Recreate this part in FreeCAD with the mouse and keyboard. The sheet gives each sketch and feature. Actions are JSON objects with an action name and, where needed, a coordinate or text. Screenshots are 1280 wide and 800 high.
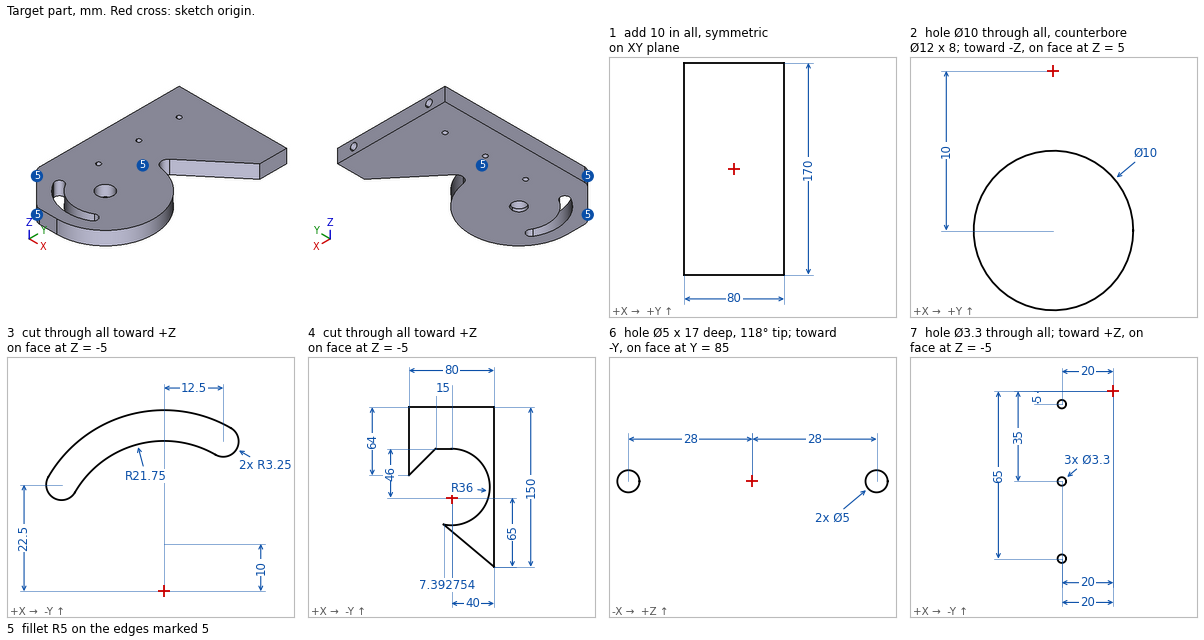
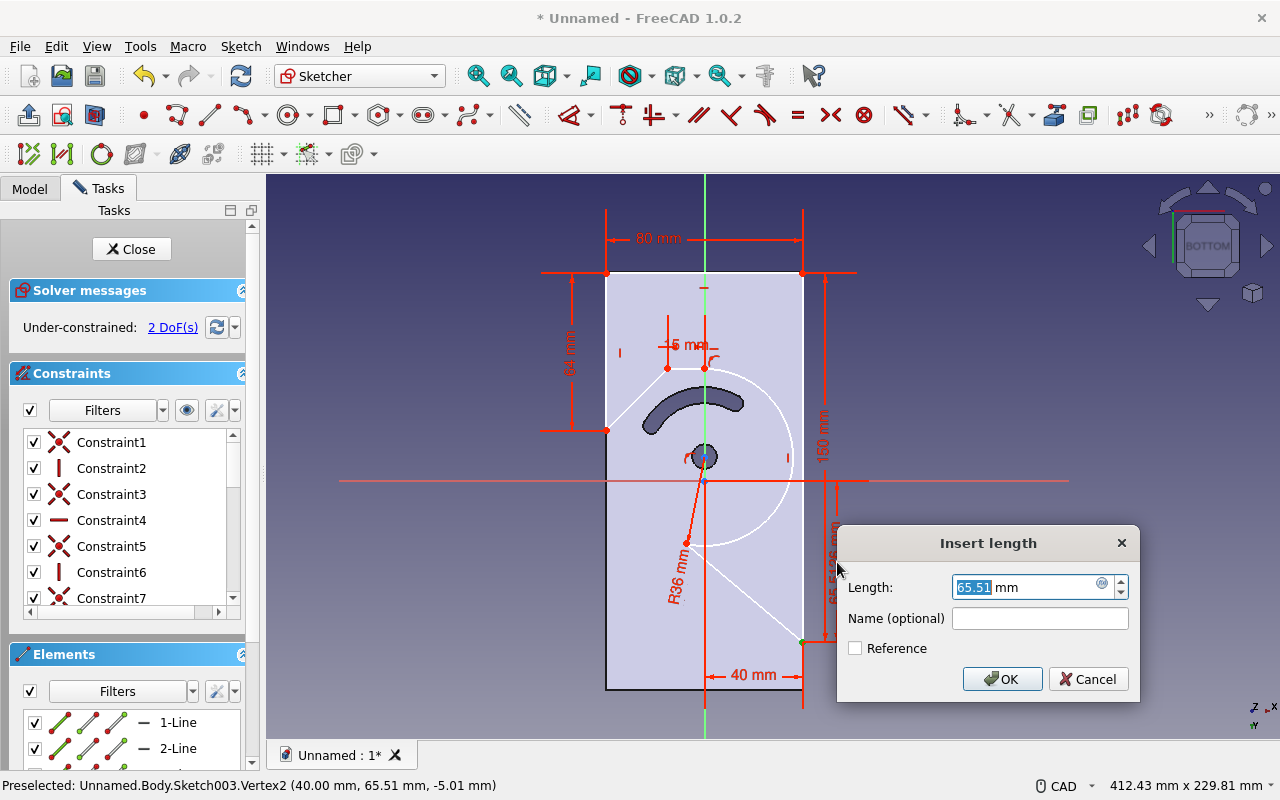
{"action": "type", "text": "65"}
{"action": "key", "text": "Return"}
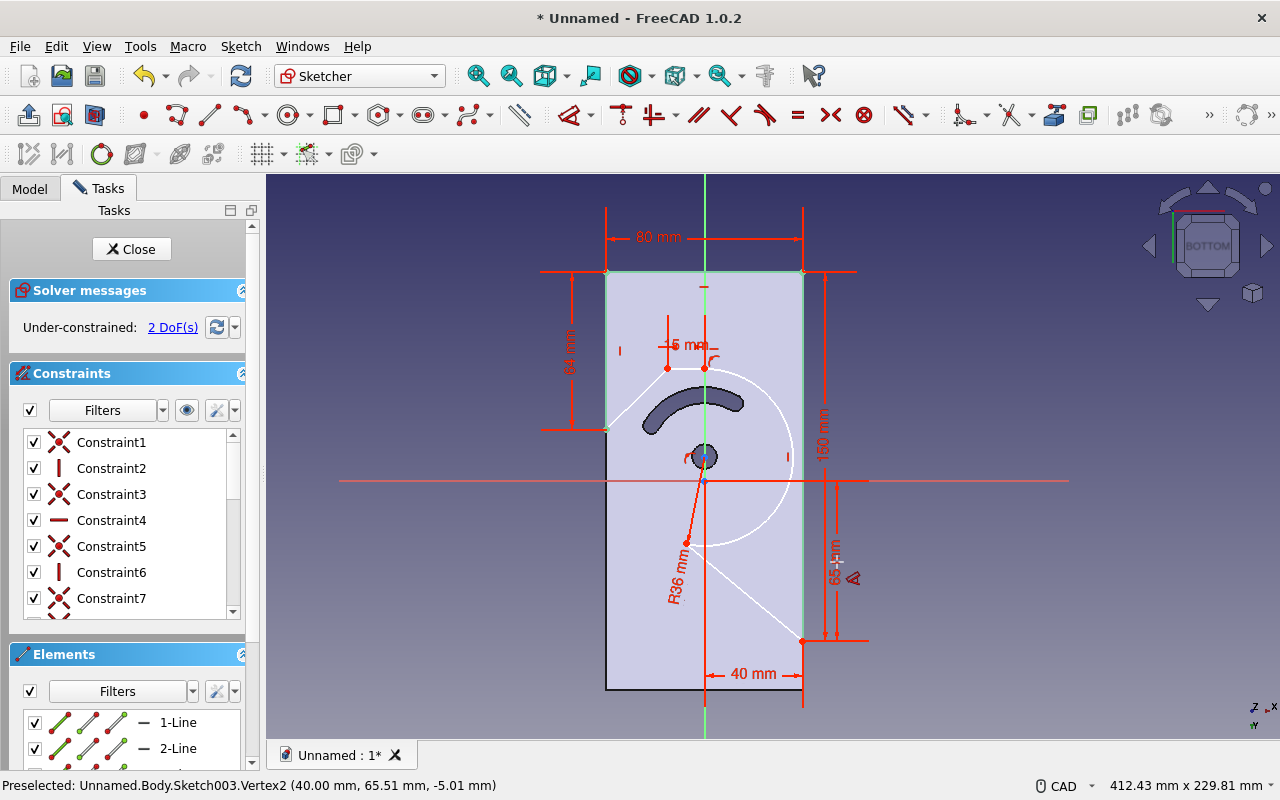
{"action": "left_click", "coordinate": [668, 369]}
{"action": "left_click", "coordinate": [634, 425]}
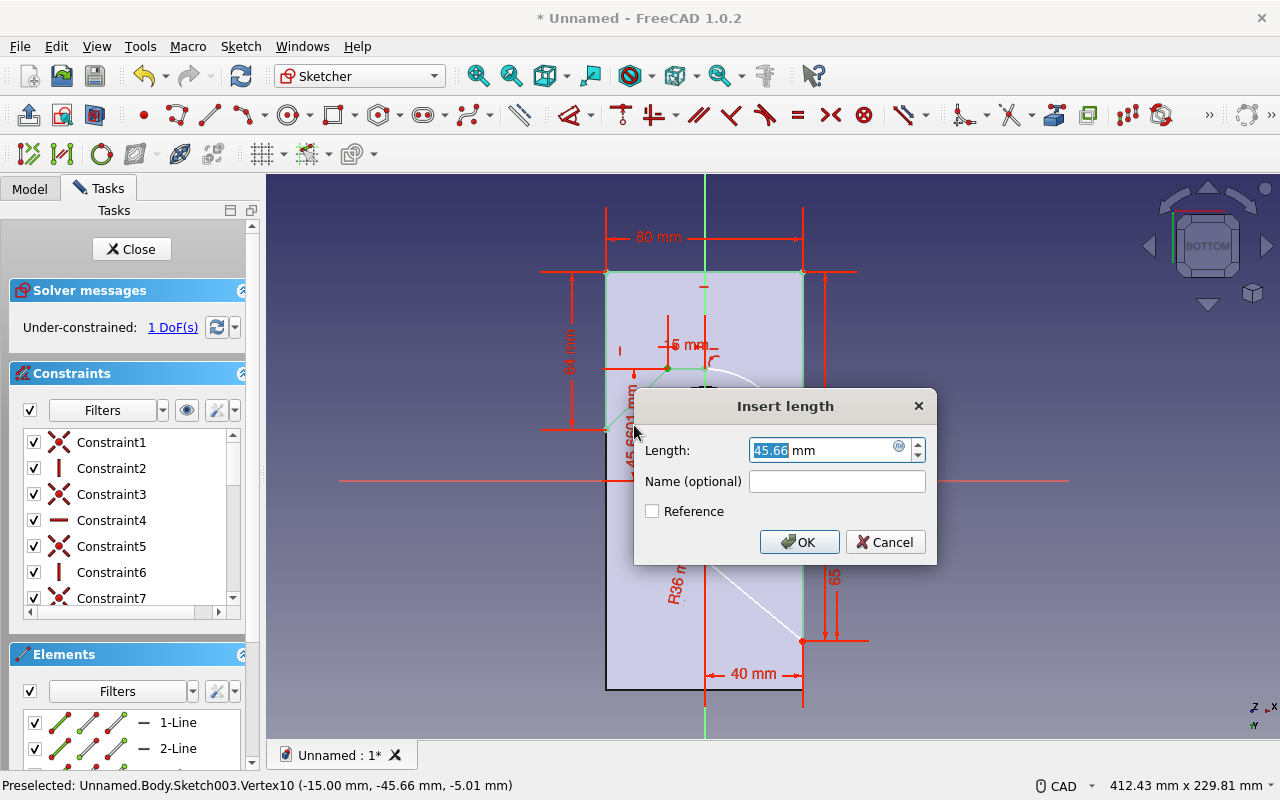
{"action": "type", "text": "46"}
{"action": "key", "text": "Return"}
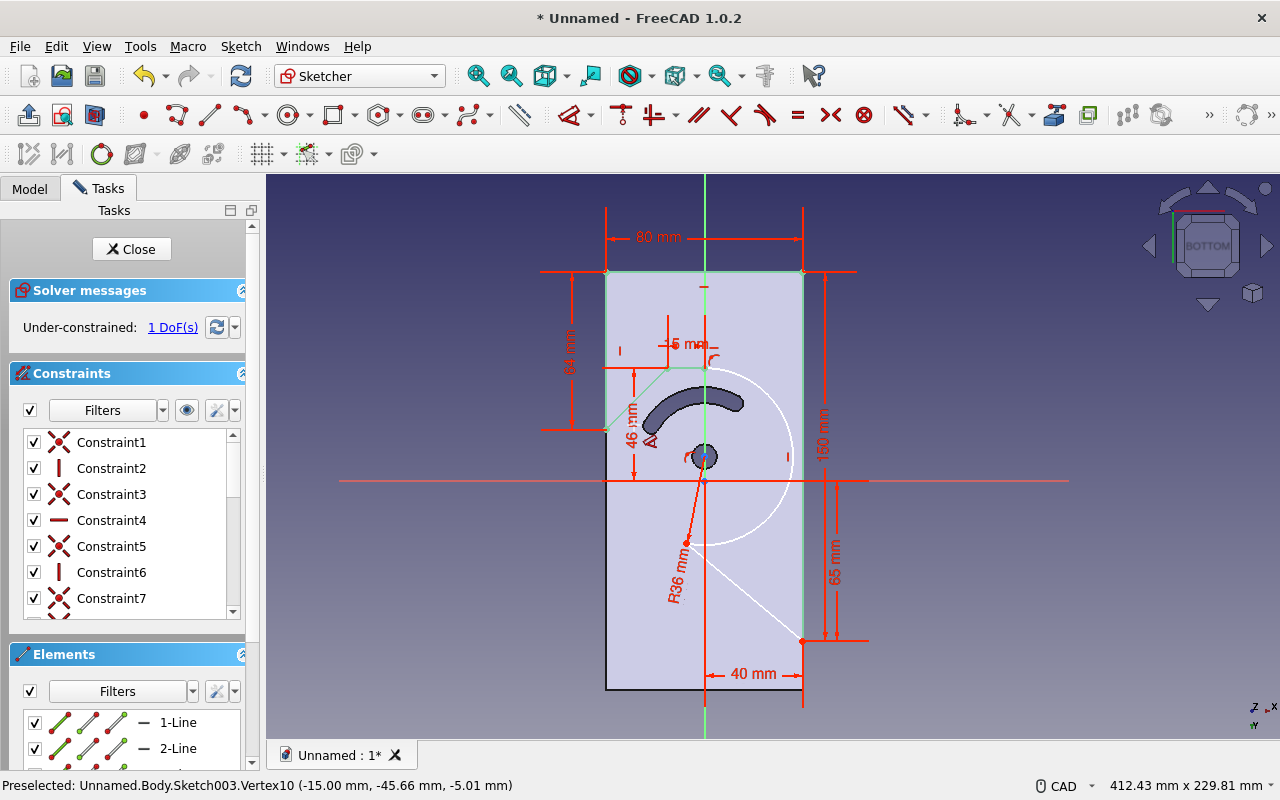
{"action": "scroll", "coordinate": [686, 543], "scroll_direction": "up", "scroll_amount": 4}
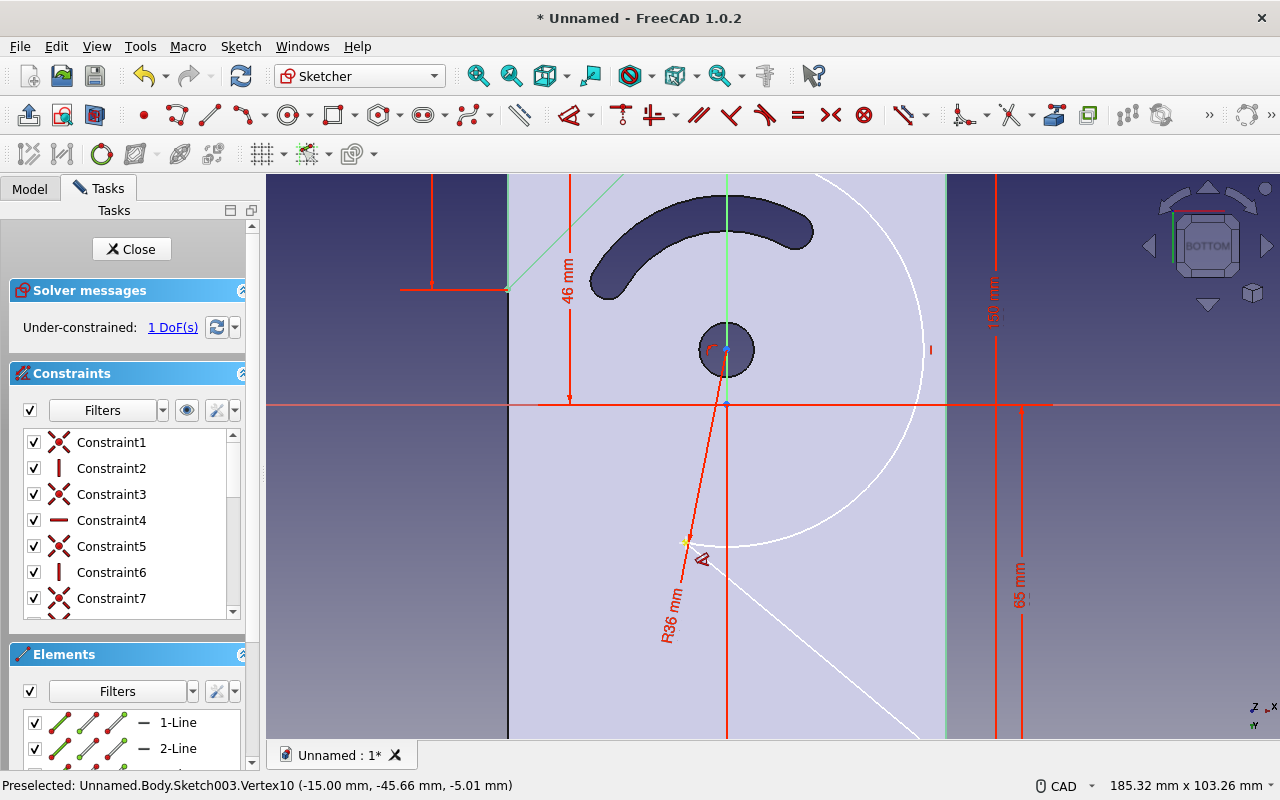
{"action": "left_click", "coordinate": [685, 543]}
{"action": "left_click", "coordinate": [697, 577]}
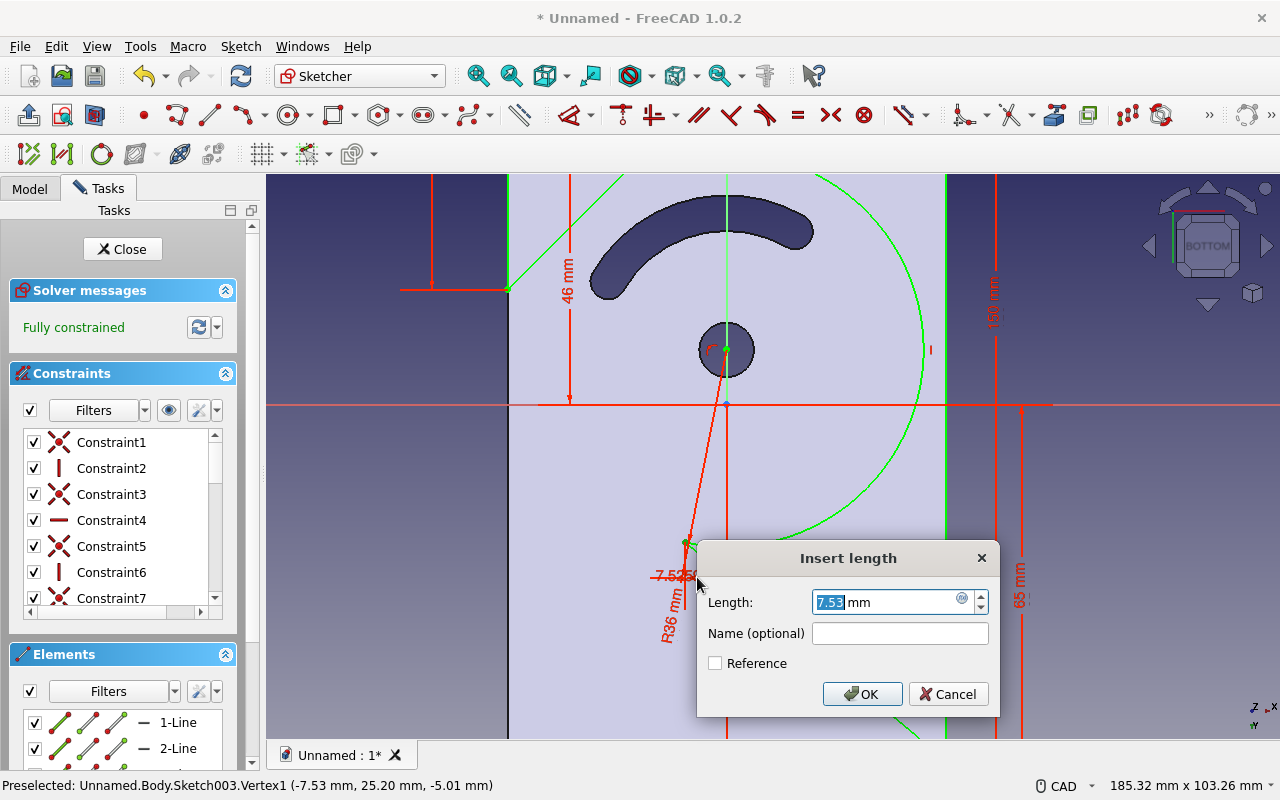
{"action": "type", "text": "7.392754"}
{"action": "key", "text": "Return"}
{"action": "key", "text": "Escape"}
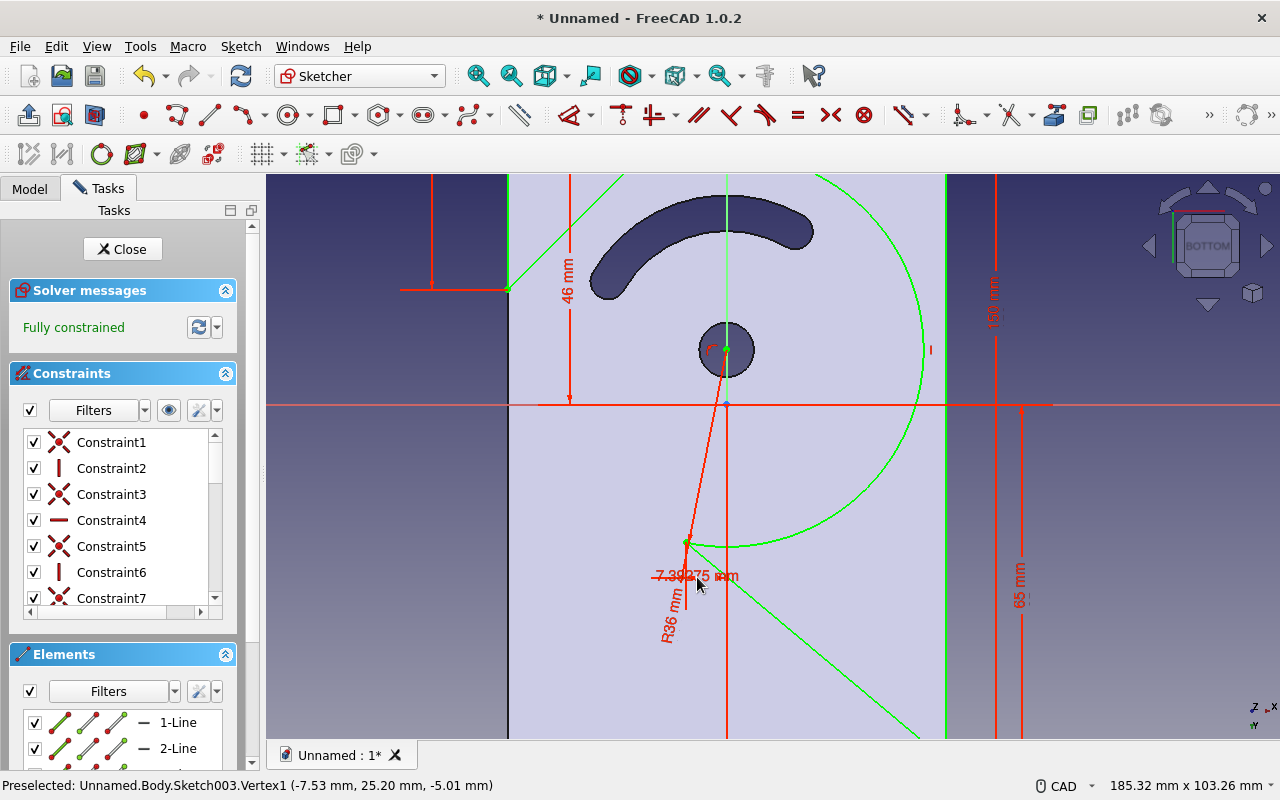
{"action": "left_click", "coordinate": [123, 249]}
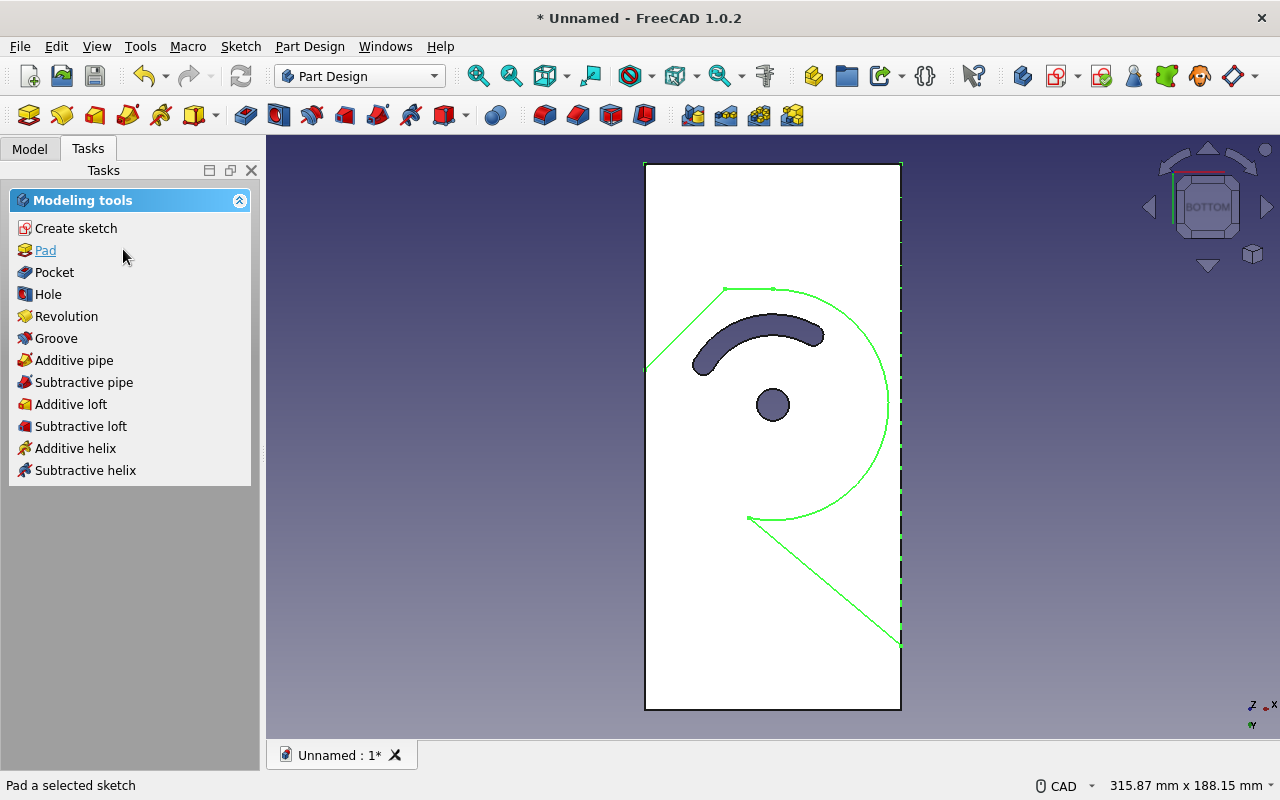
{"action": "left_click", "coordinate": [246, 116]}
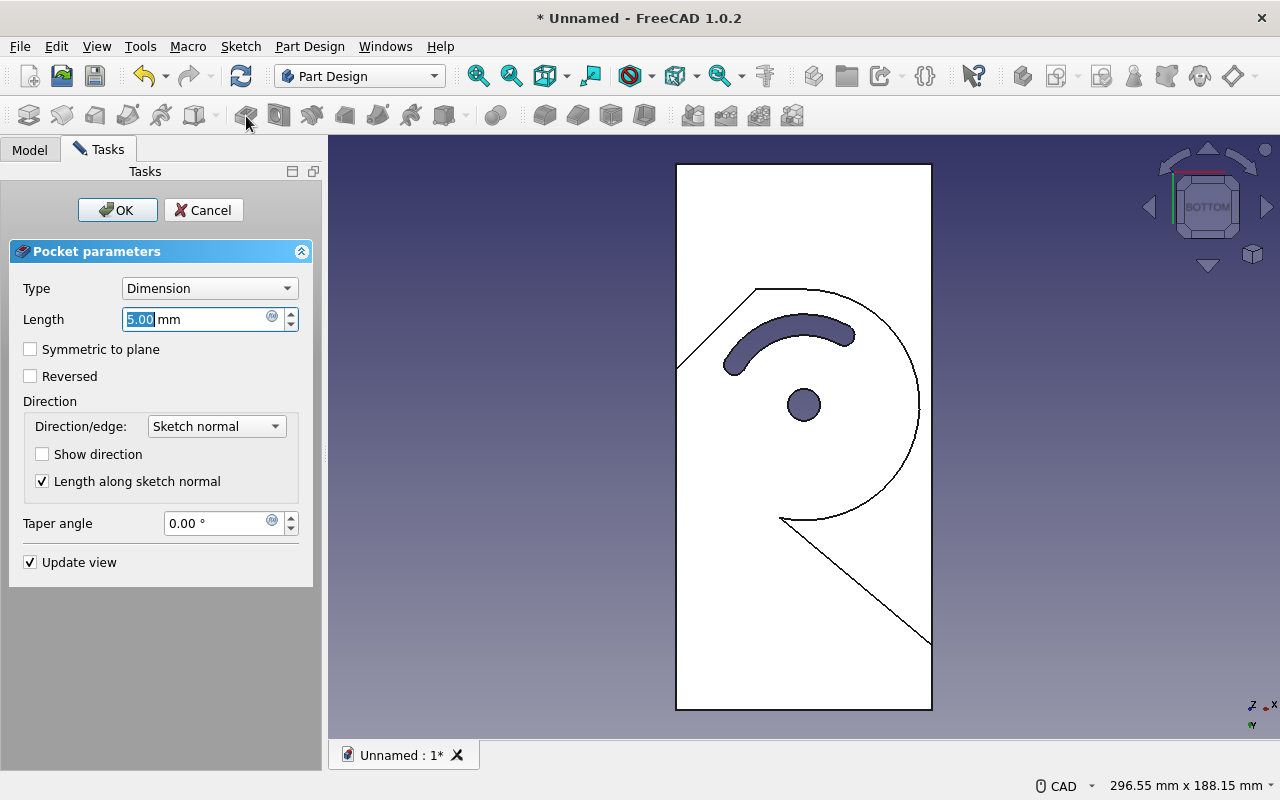
{"action": "left_click", "coordinate": [210, 288]}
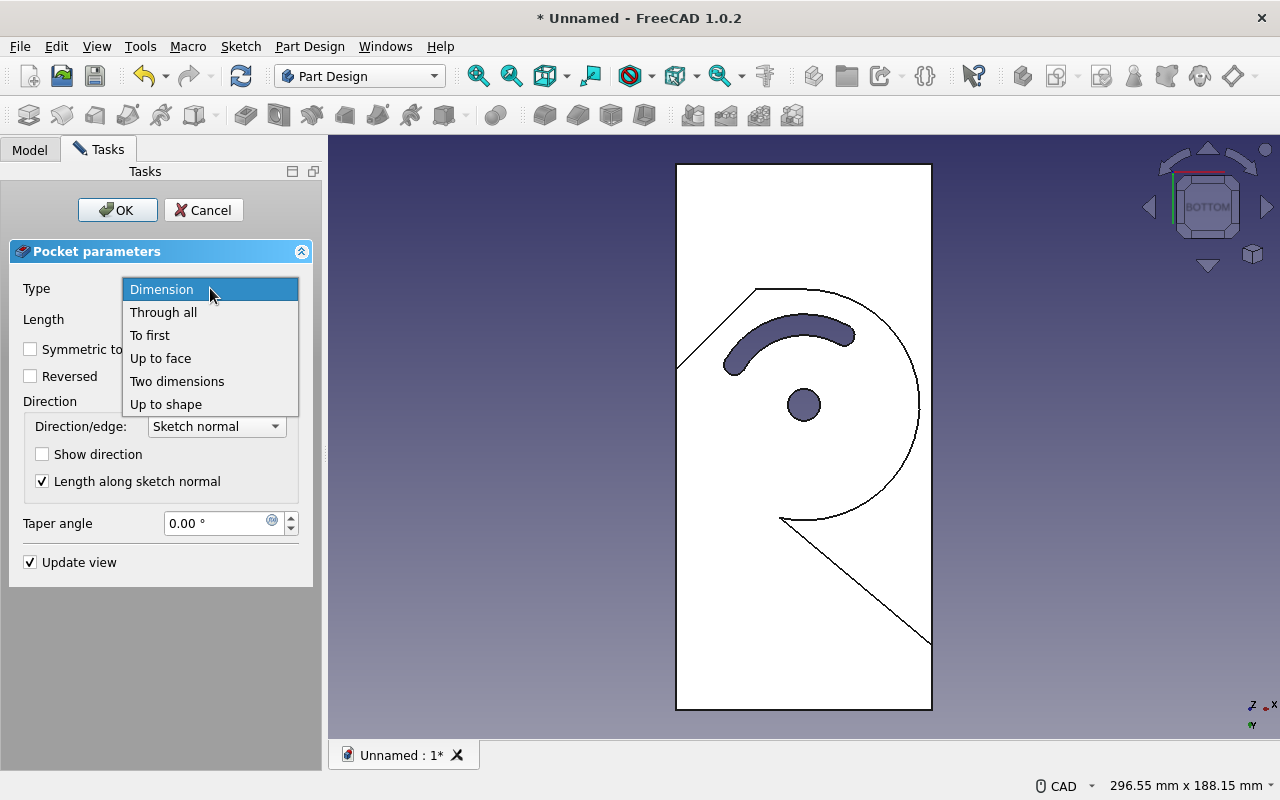
{"action": "left_click", "coordinate": [208, 312]}